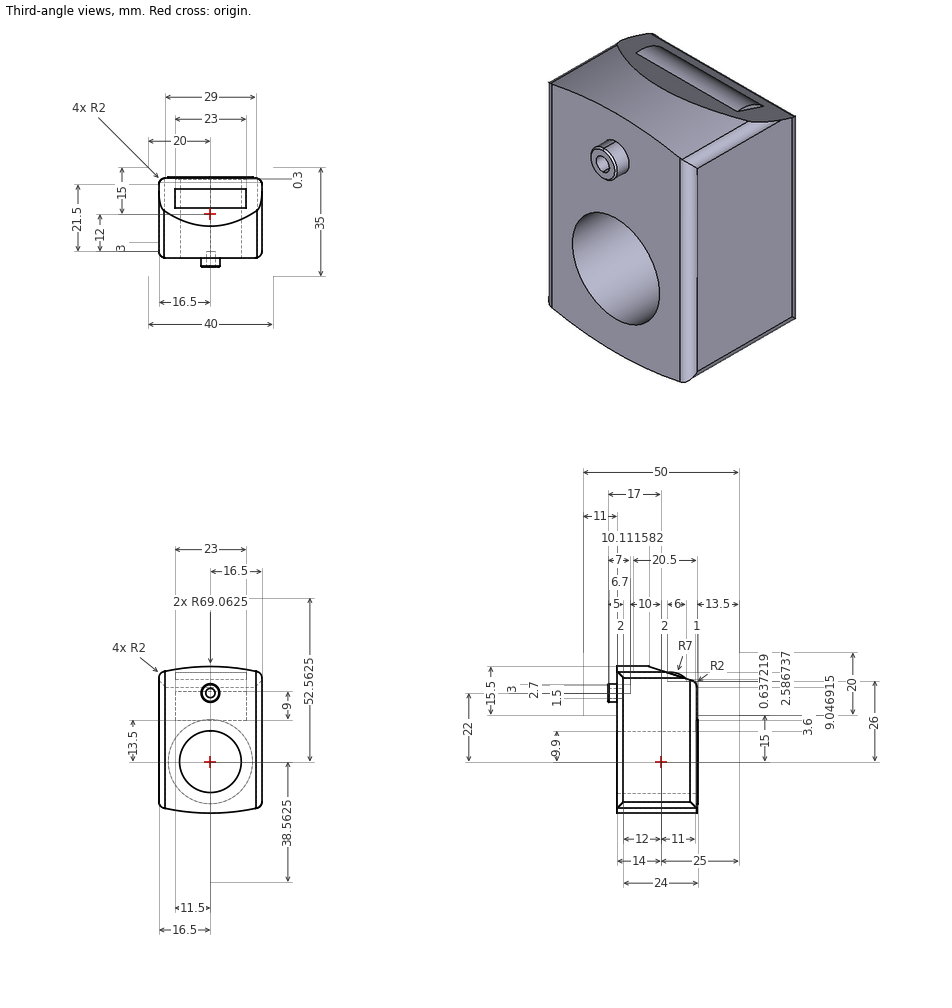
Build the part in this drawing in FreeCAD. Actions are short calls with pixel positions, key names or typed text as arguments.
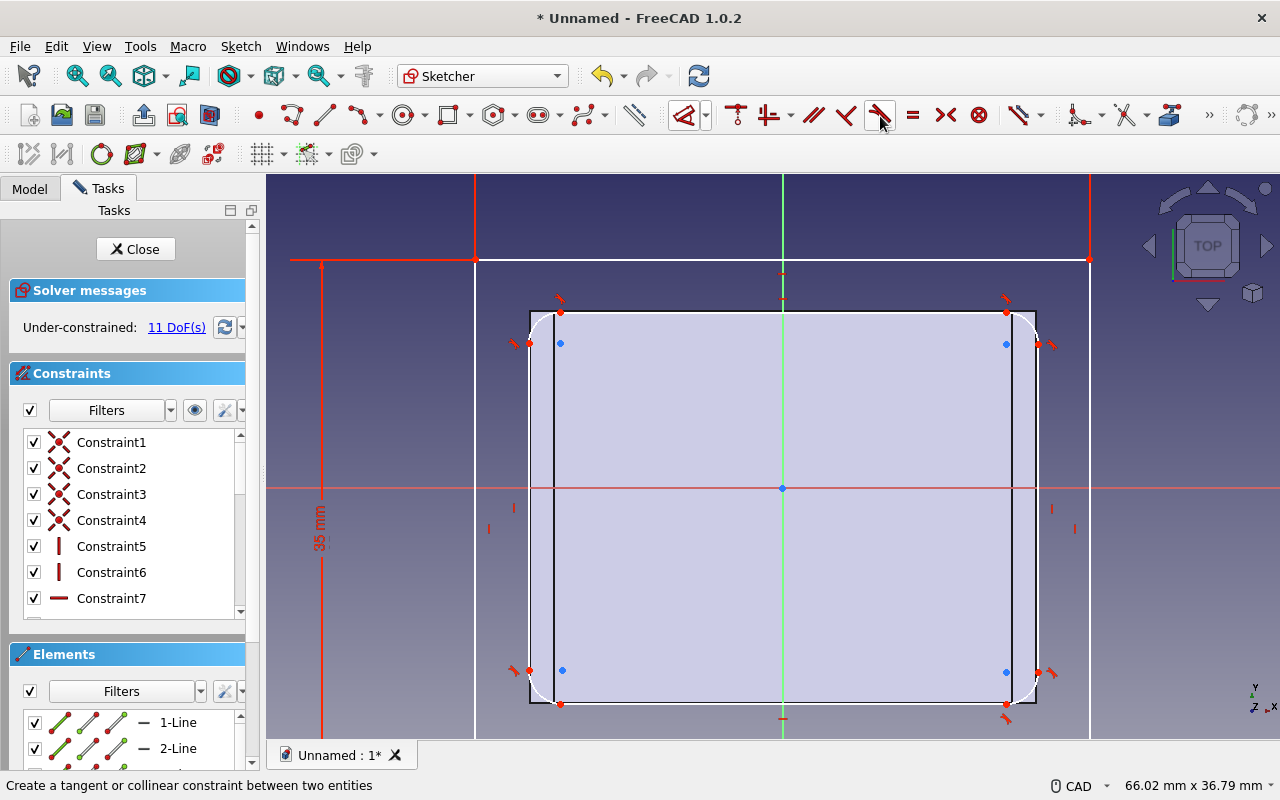
click(872, 704)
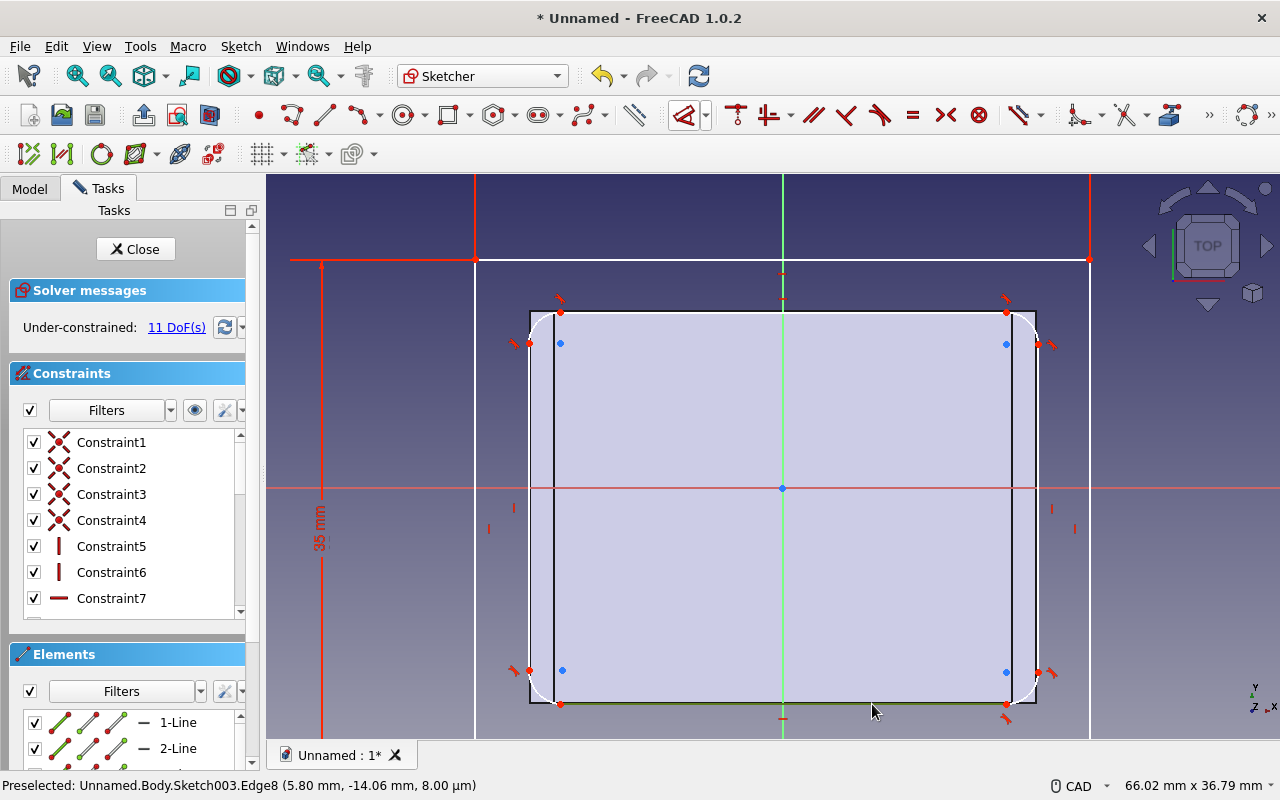
click(532, 685)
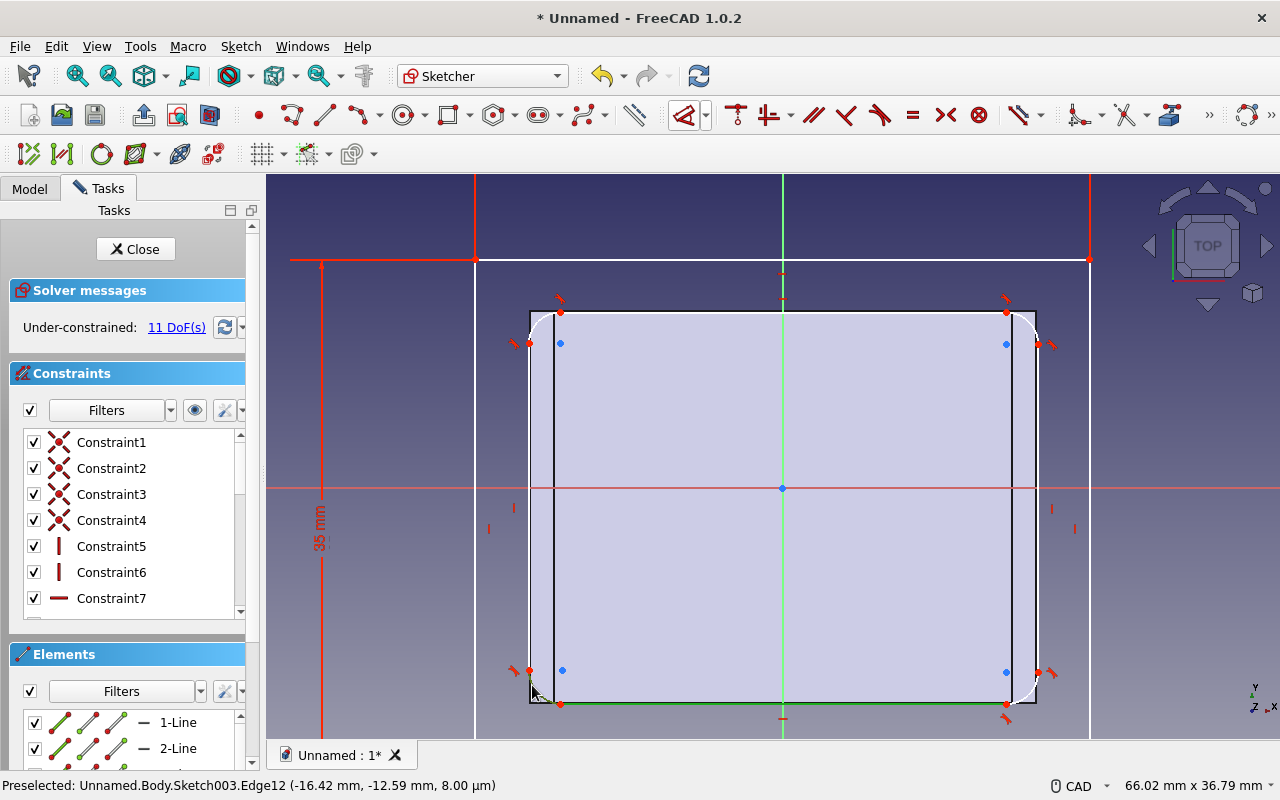
click(880, 116)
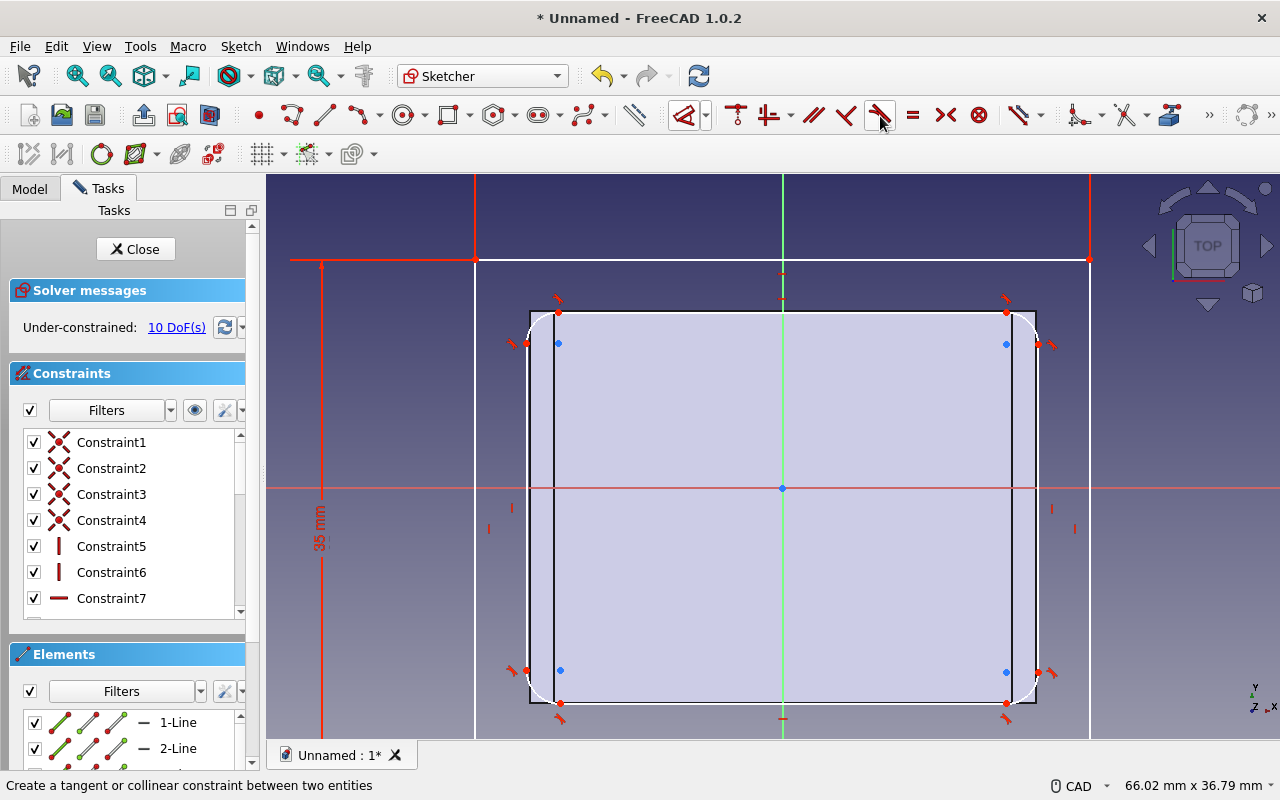
click(544, 316)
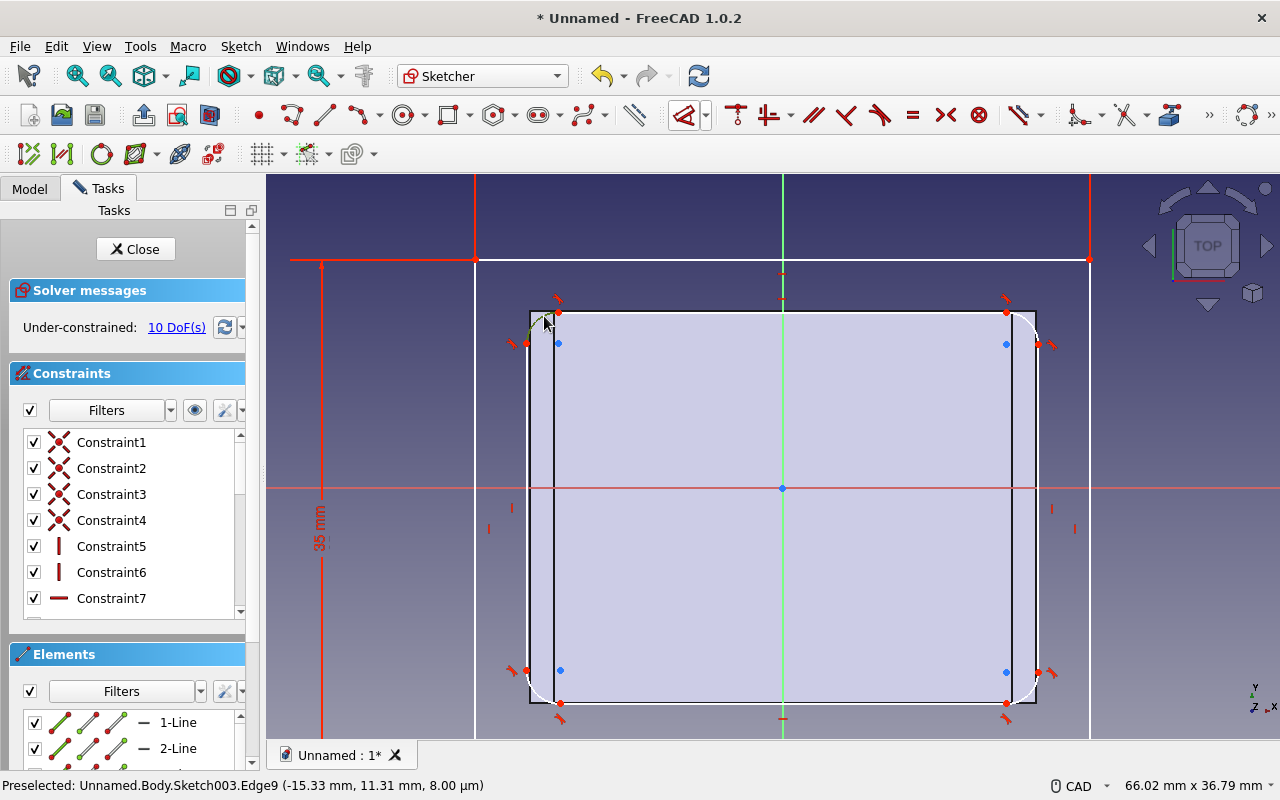
click(1035, 330)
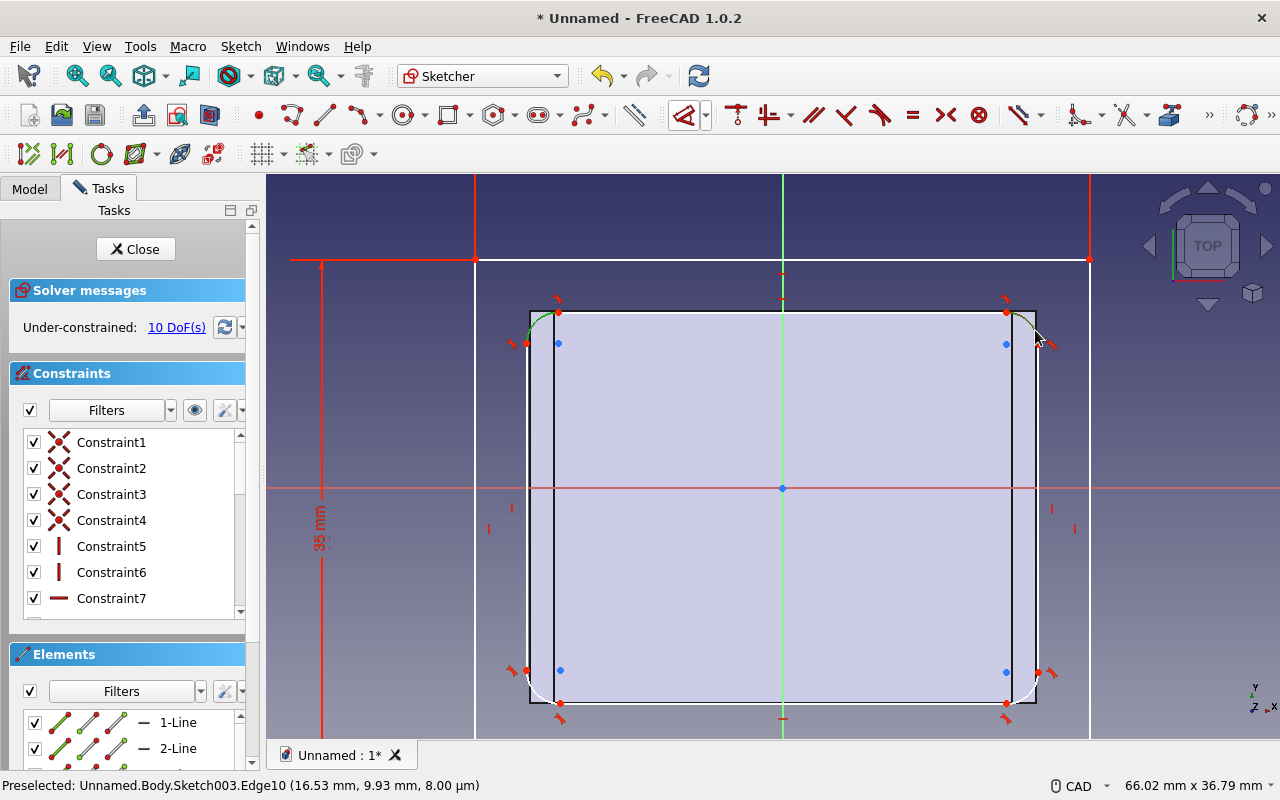
click(1021, 700)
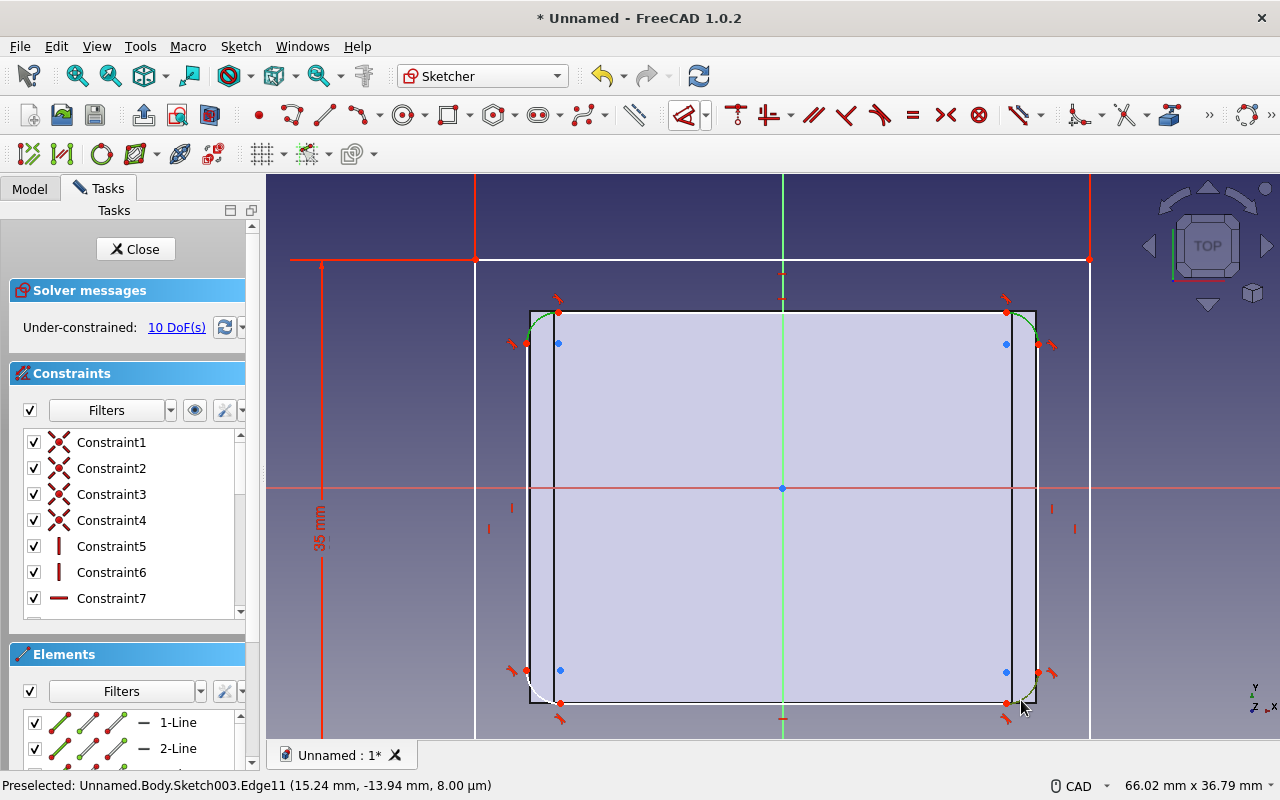
click(531, 686)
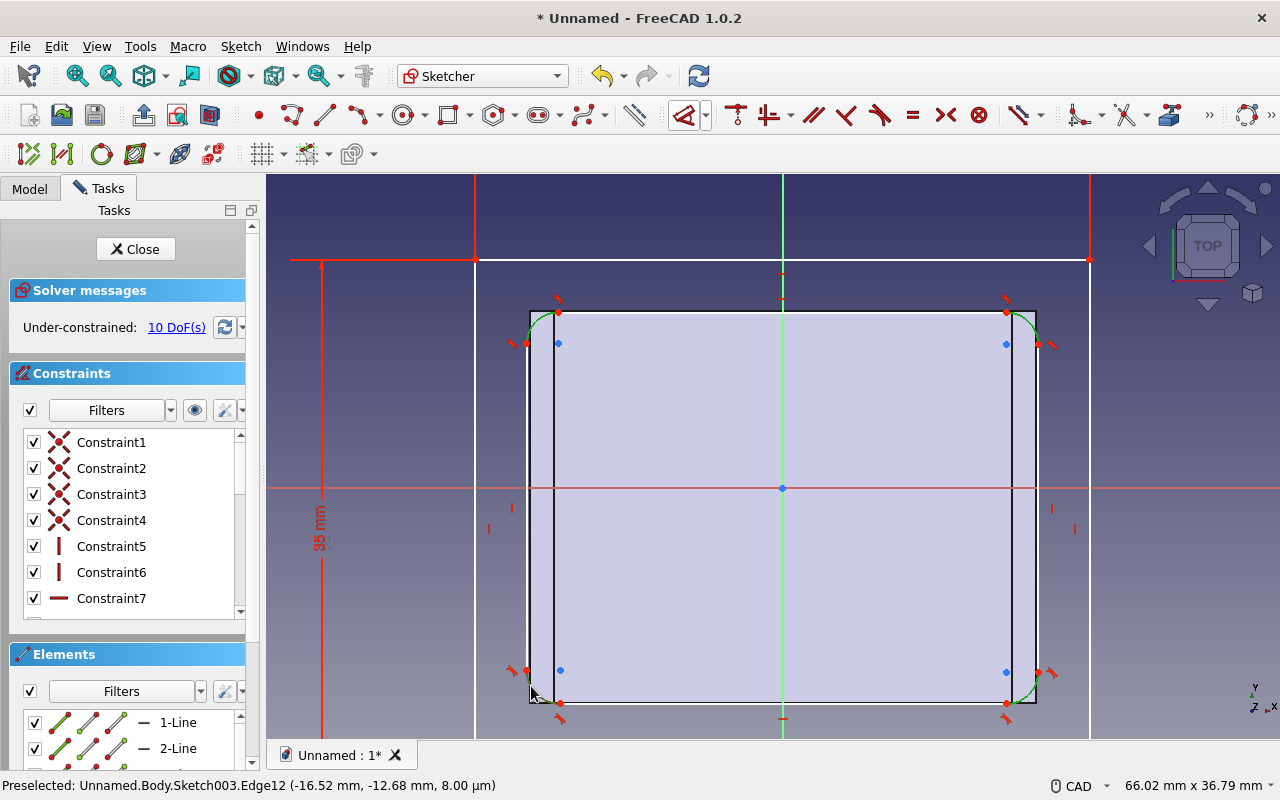
click(913, 116)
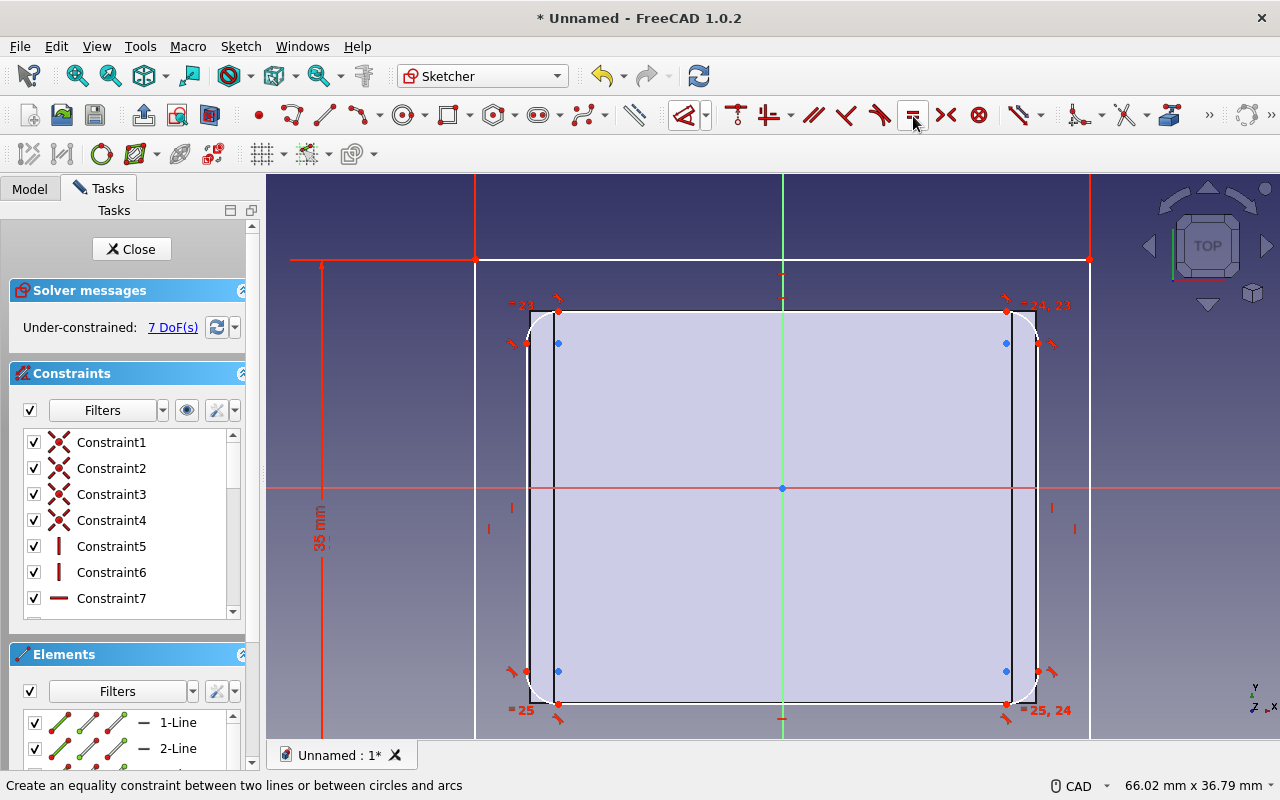
scroll(544, 315, up, 2)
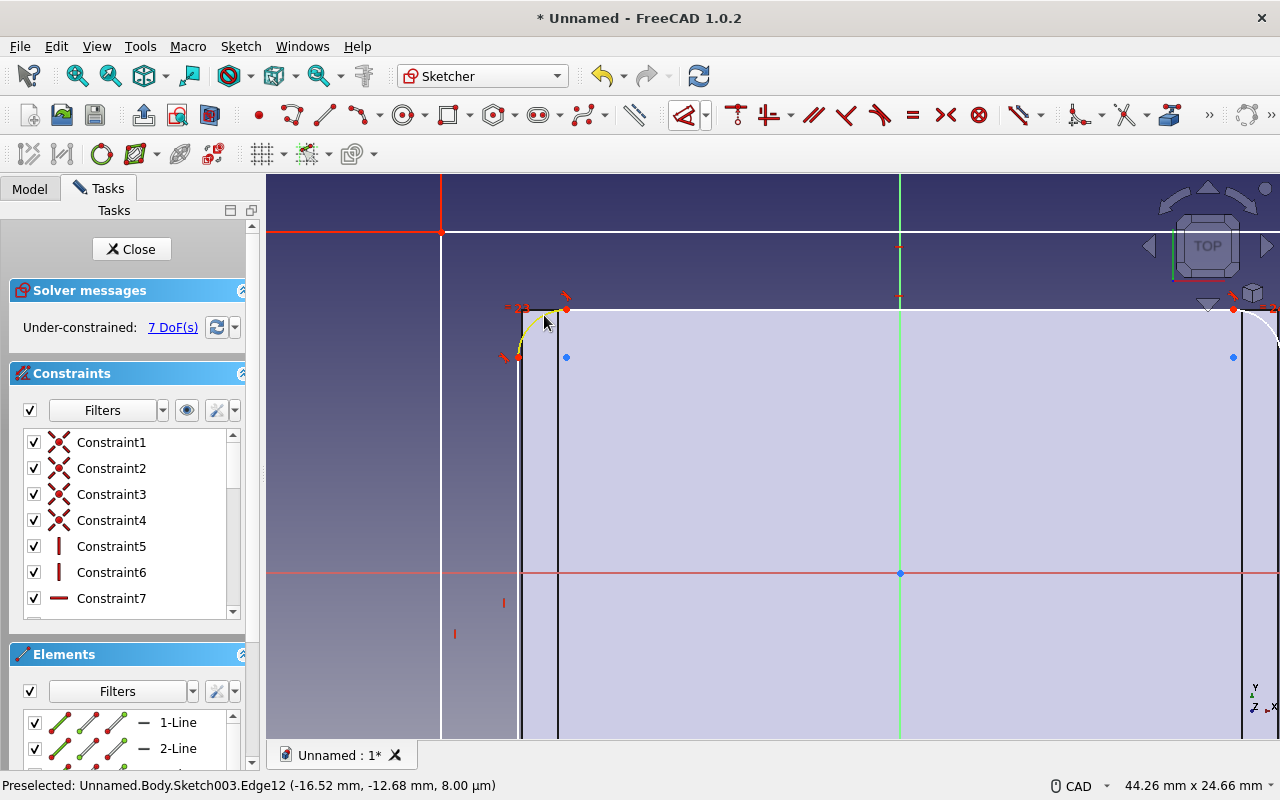
click(544, 315)